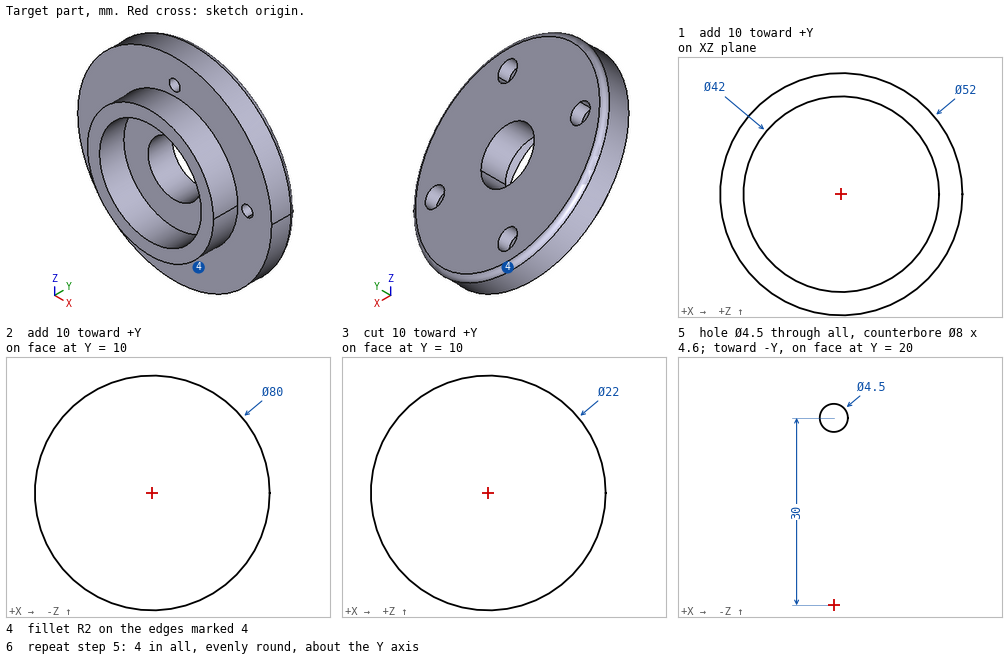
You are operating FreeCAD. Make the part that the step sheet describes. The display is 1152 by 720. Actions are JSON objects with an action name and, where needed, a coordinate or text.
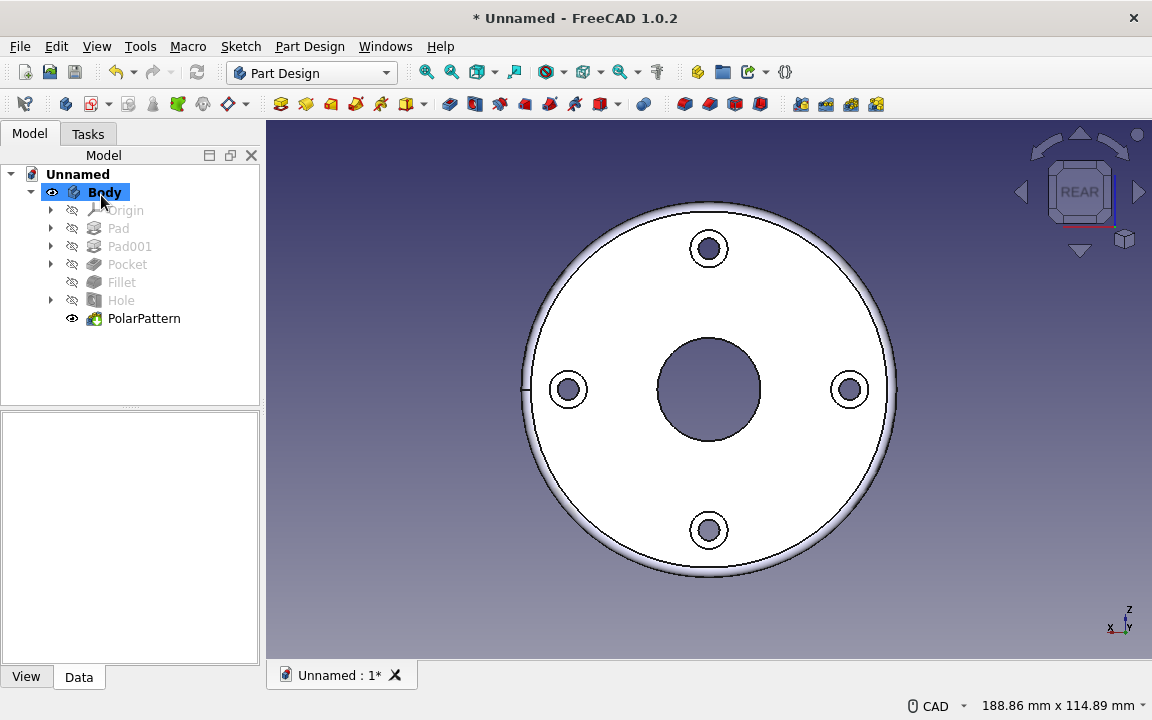
{"action": "key", "text": "0"}